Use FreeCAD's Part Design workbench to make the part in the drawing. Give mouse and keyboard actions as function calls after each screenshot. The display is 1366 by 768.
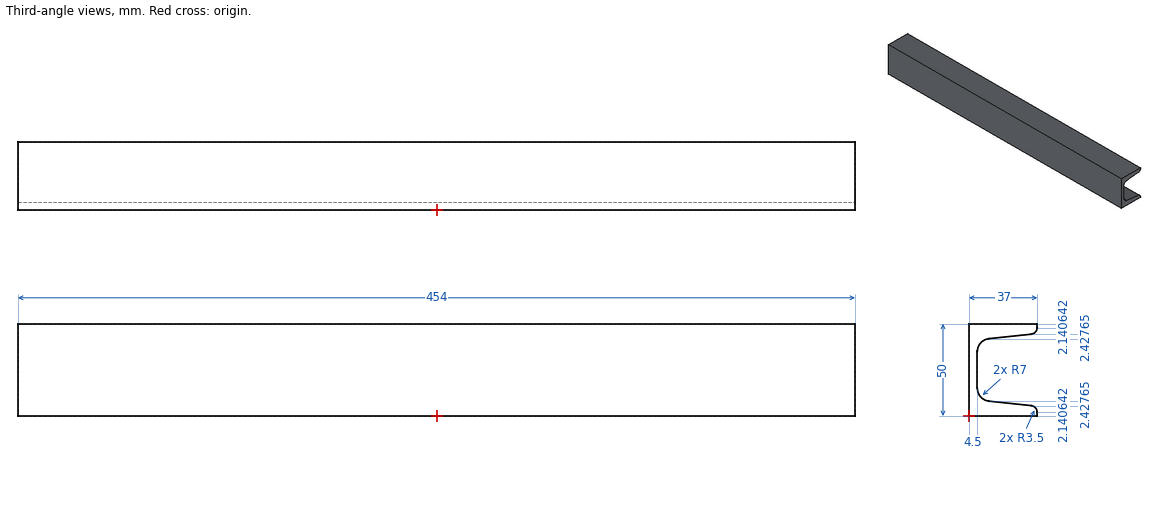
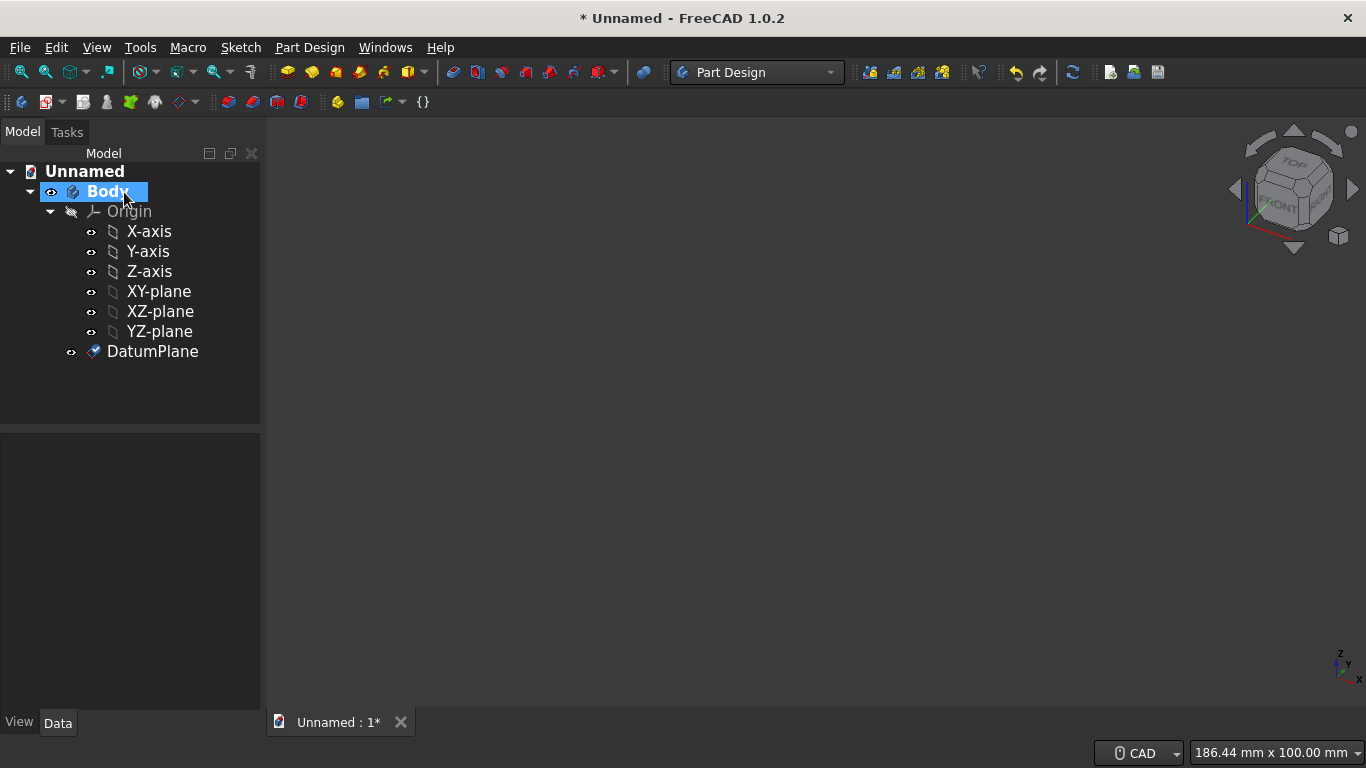
click(116, 352)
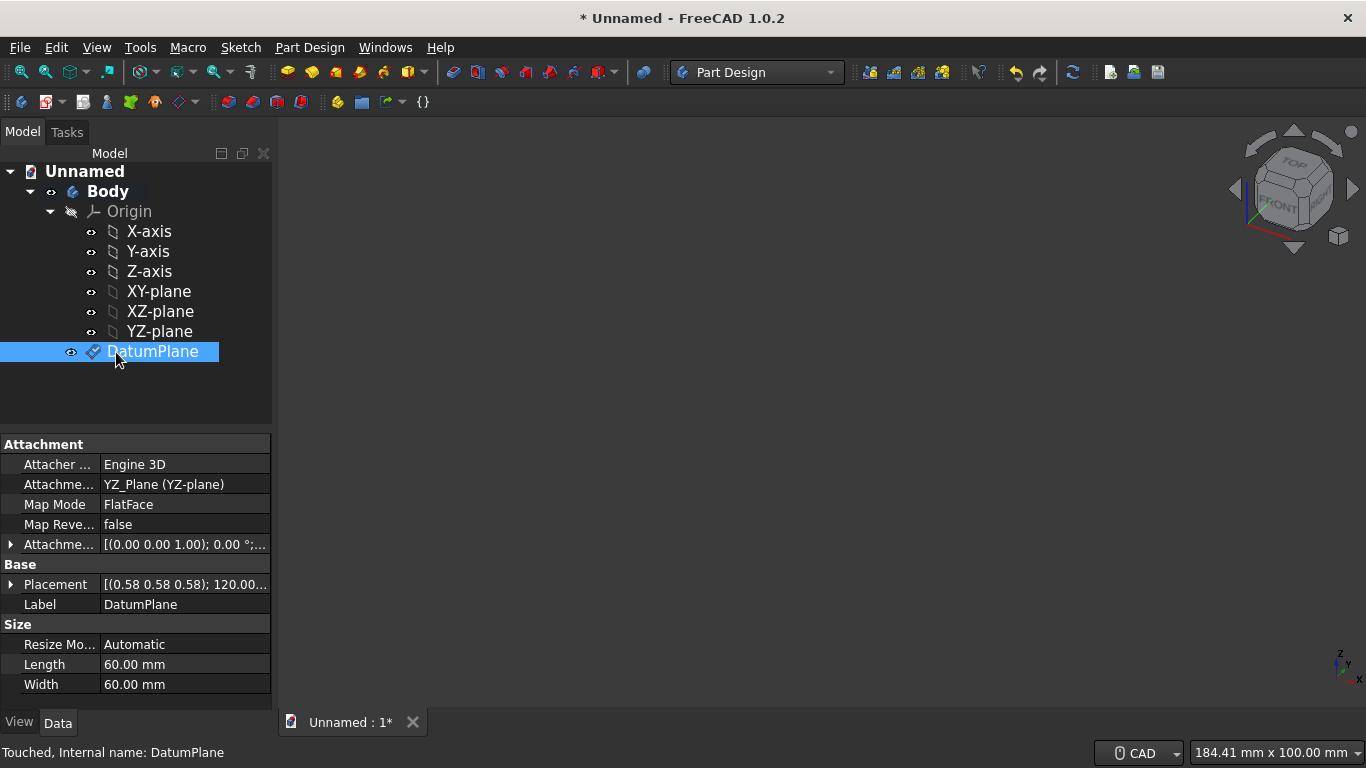
click(46, 102)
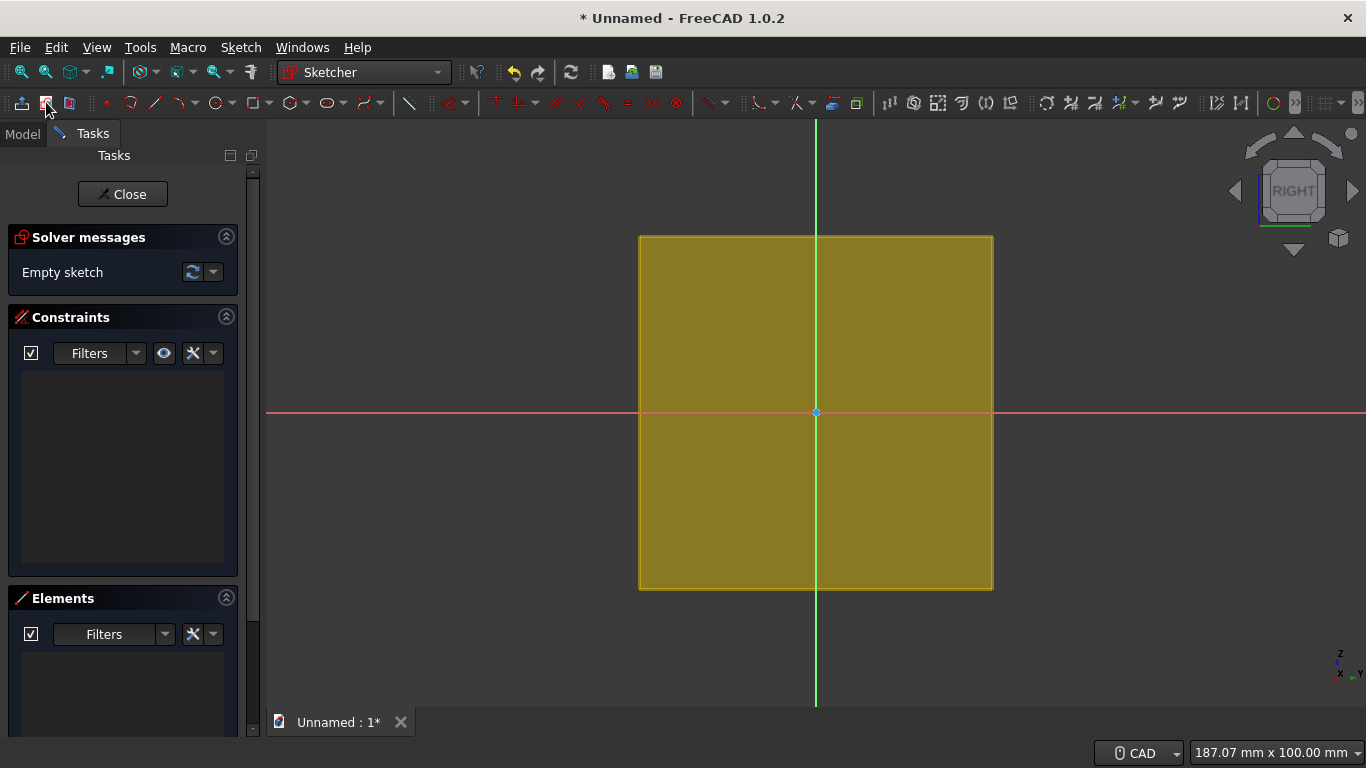
scroll(294, 679, down, 1)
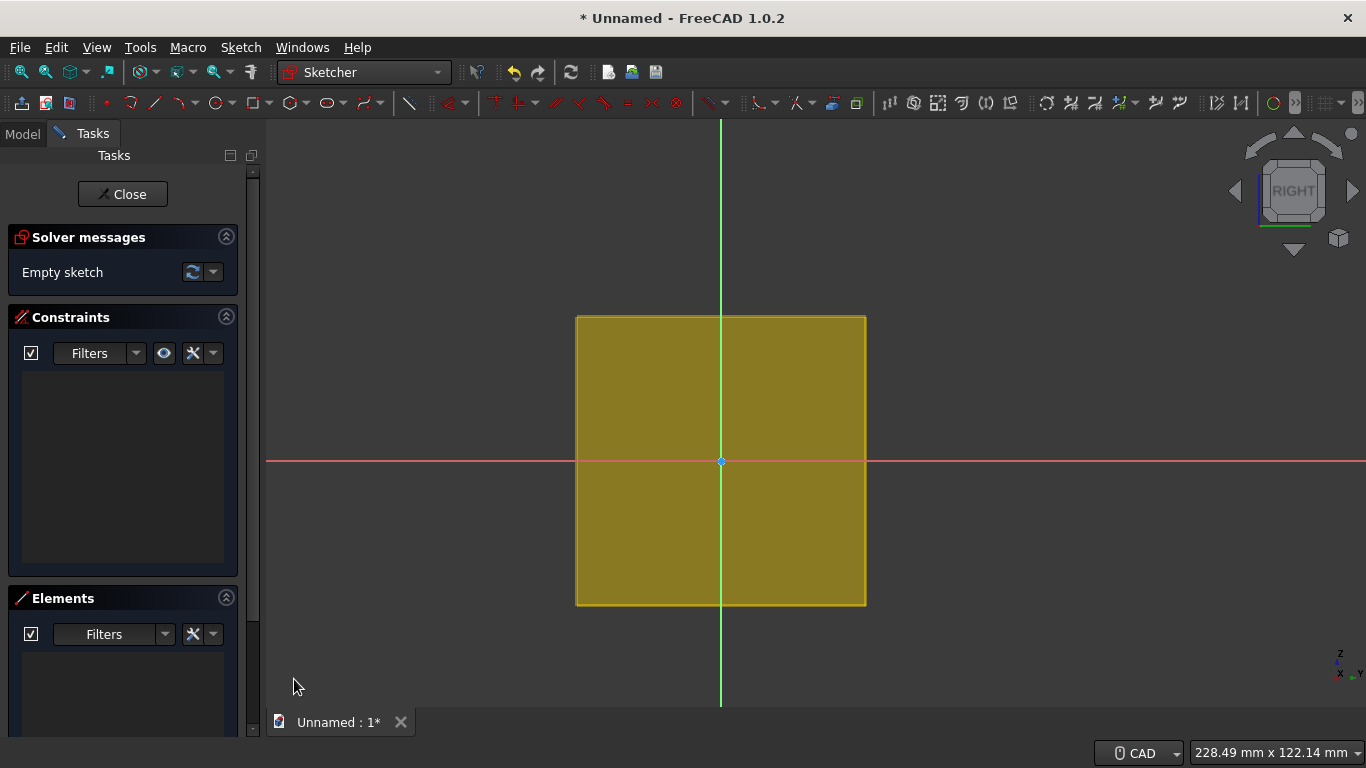
scroll(938, 195, up, 2)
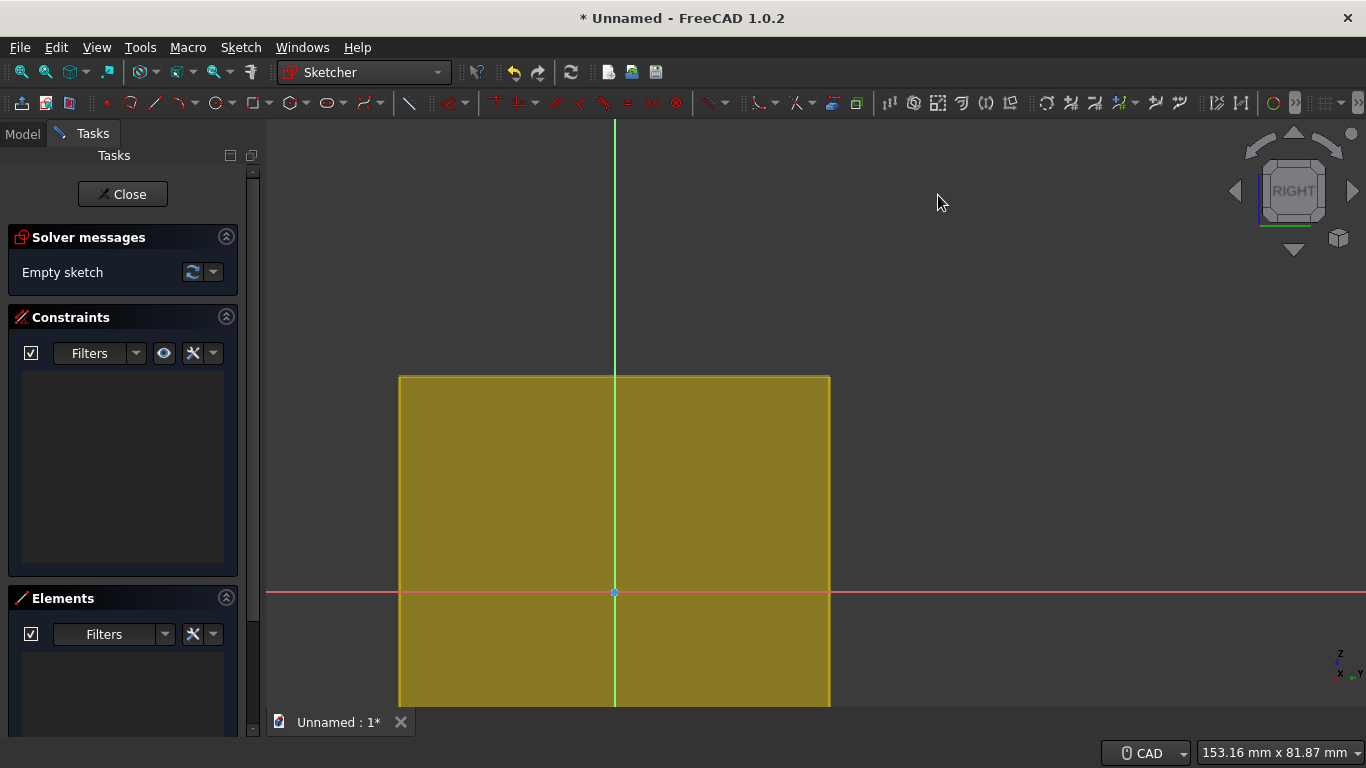
click(156, 104)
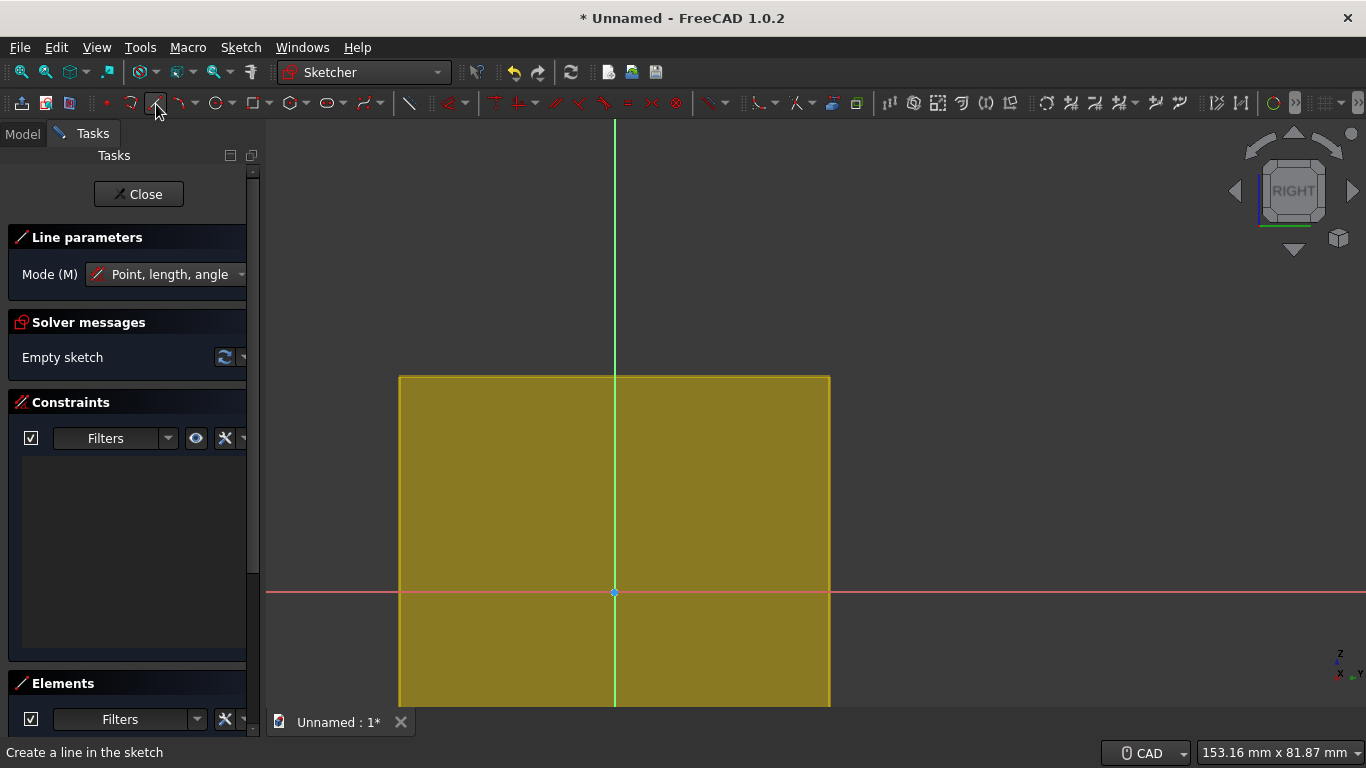
click(858, 552)
click(692, 535)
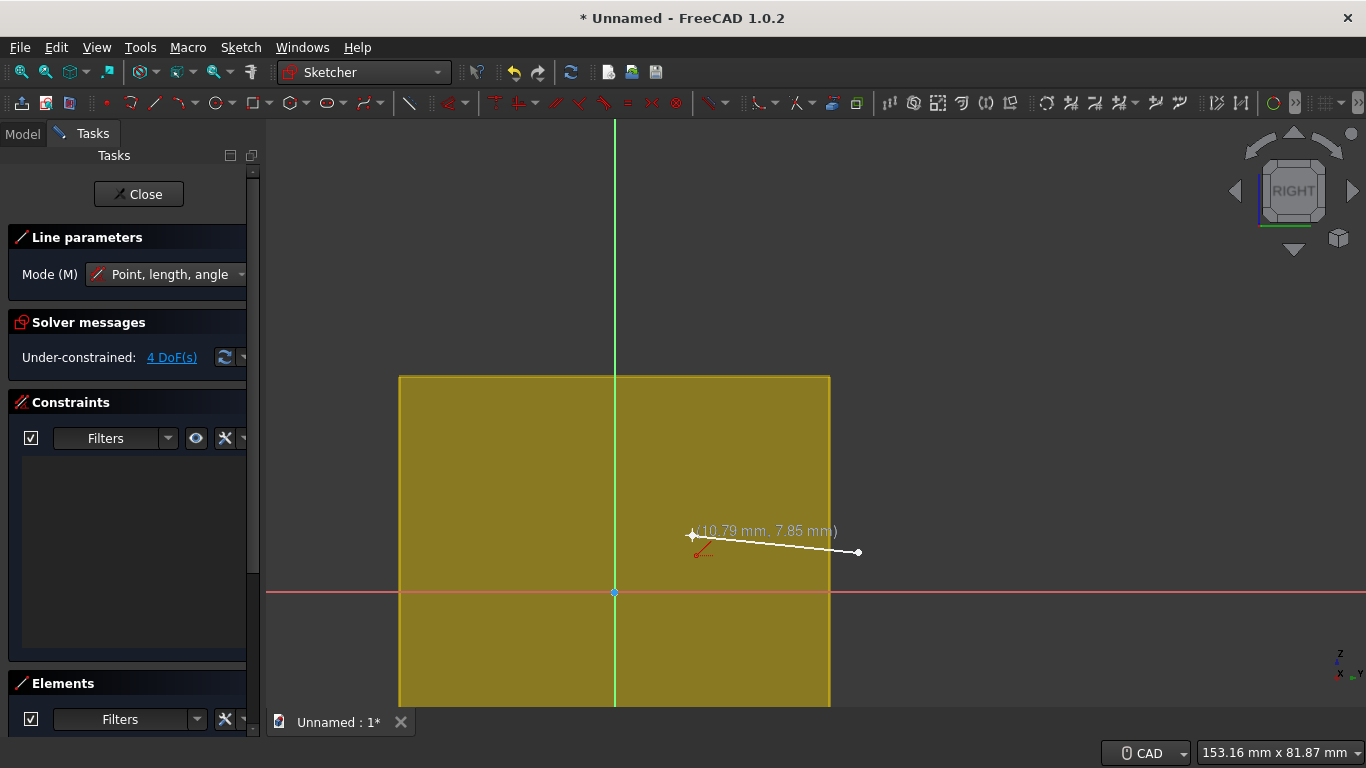
click(647, 485)
click(647, 341)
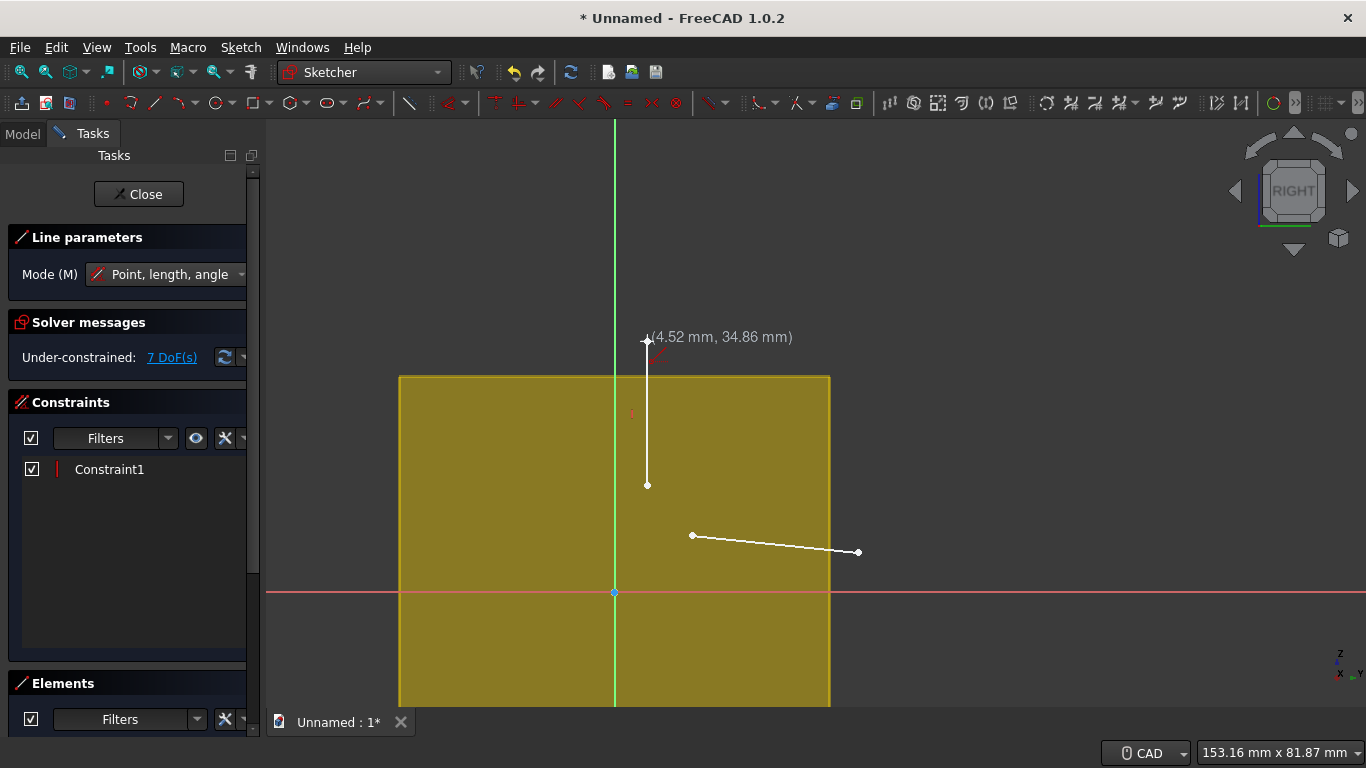
click(692, 291)
click(858, 274)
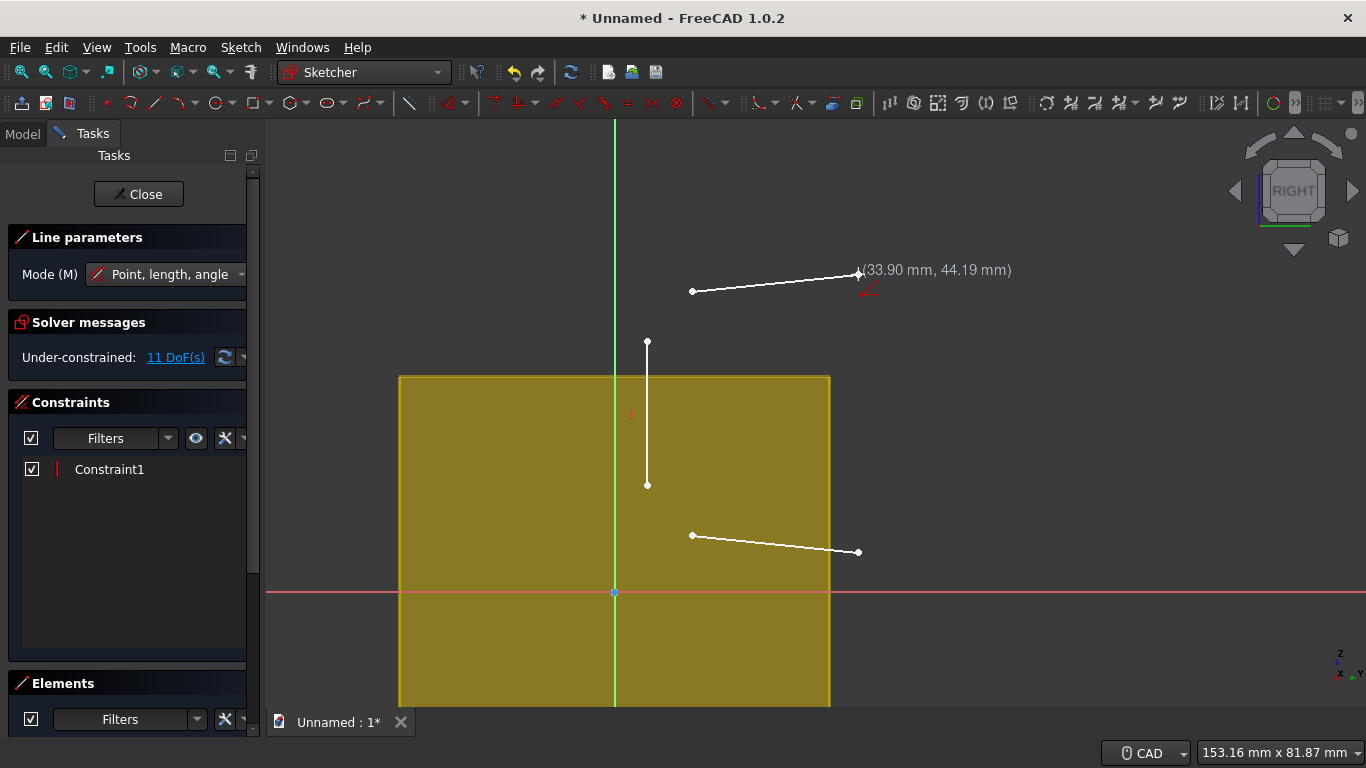
click(132, 104)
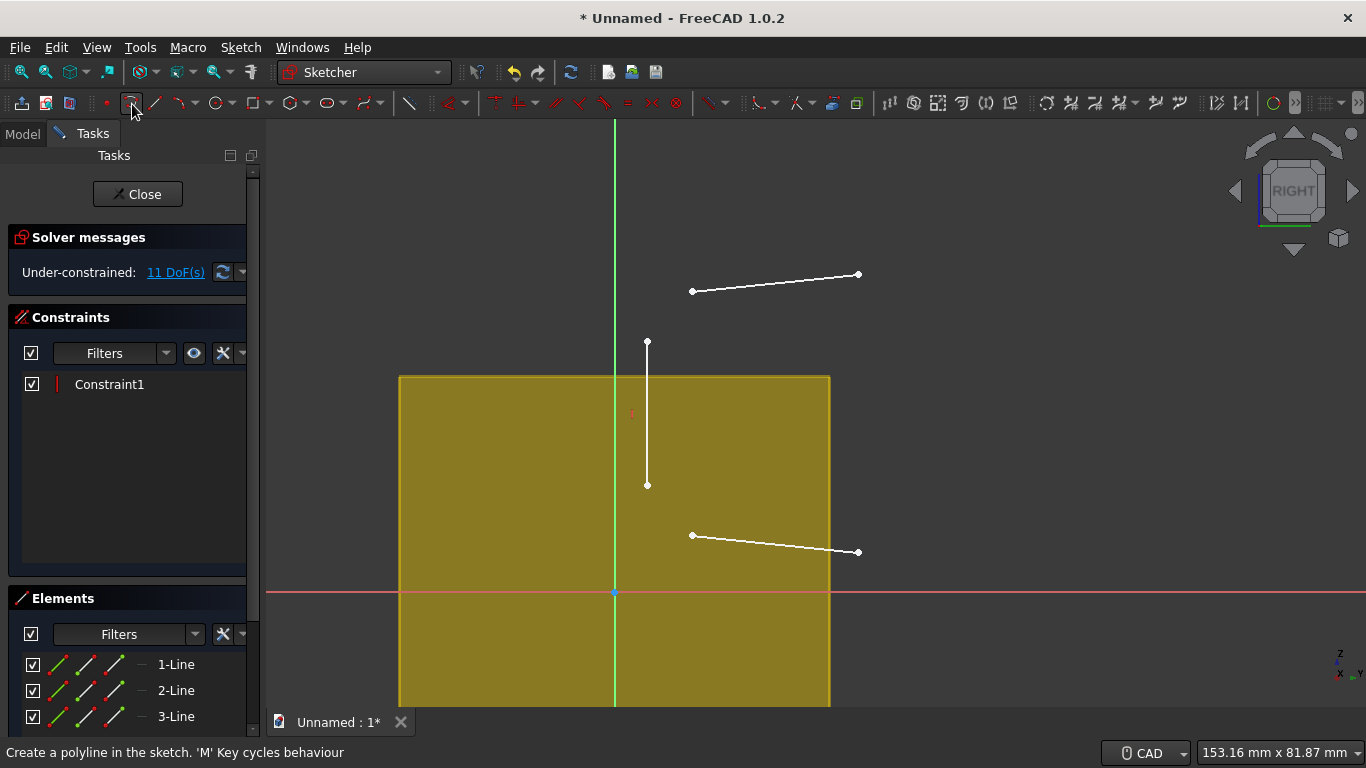
click(880, 249)
click(880, 233)
click(615, 233)
click(615, 592)
click(880, 583)
click(880, 577)
right_click(880, 577)